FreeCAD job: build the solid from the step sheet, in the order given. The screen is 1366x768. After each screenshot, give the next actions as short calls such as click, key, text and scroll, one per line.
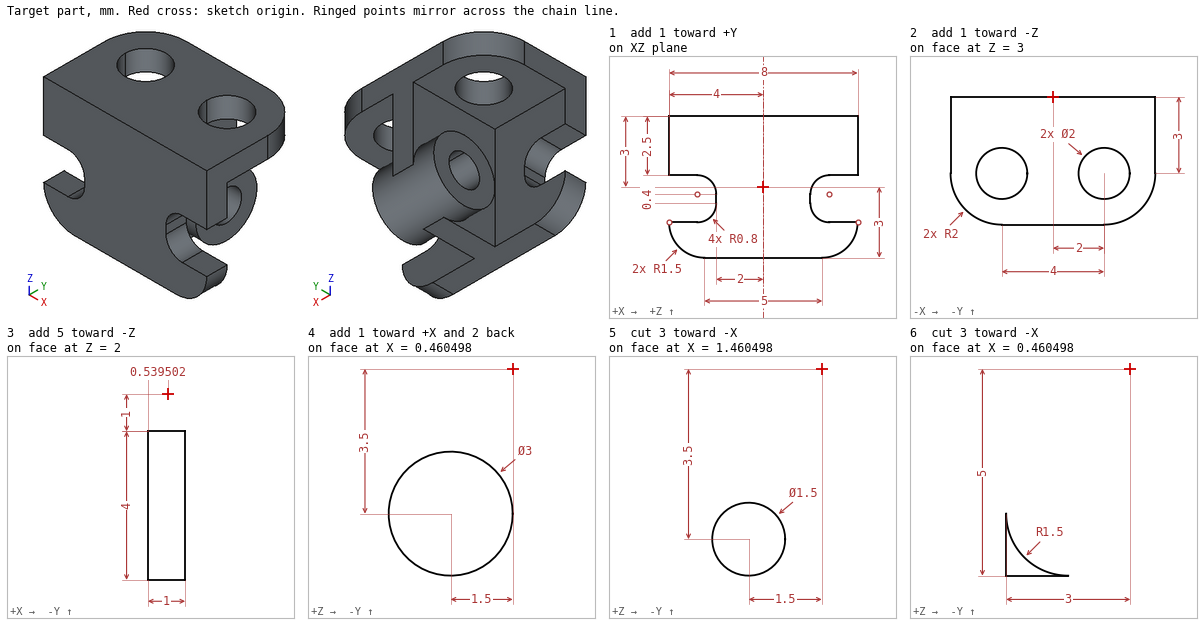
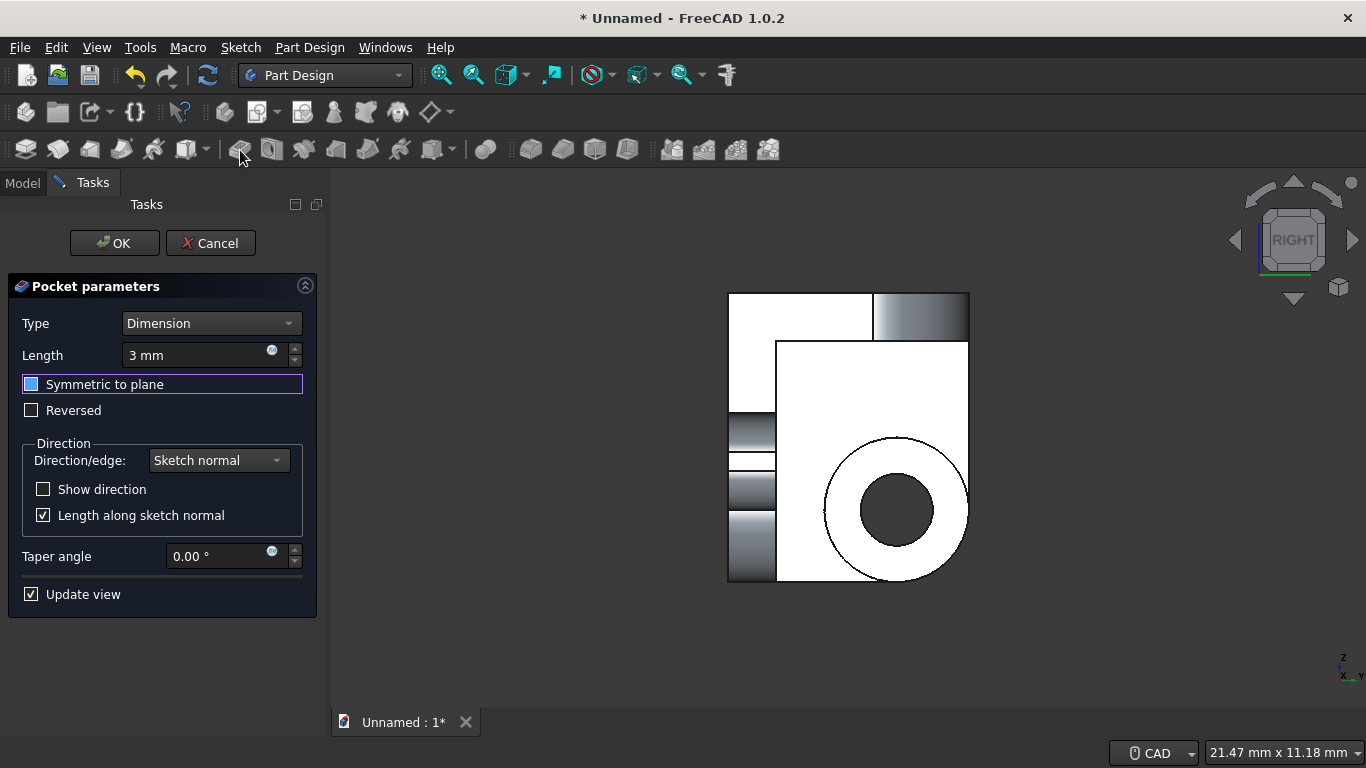
click(115, 243)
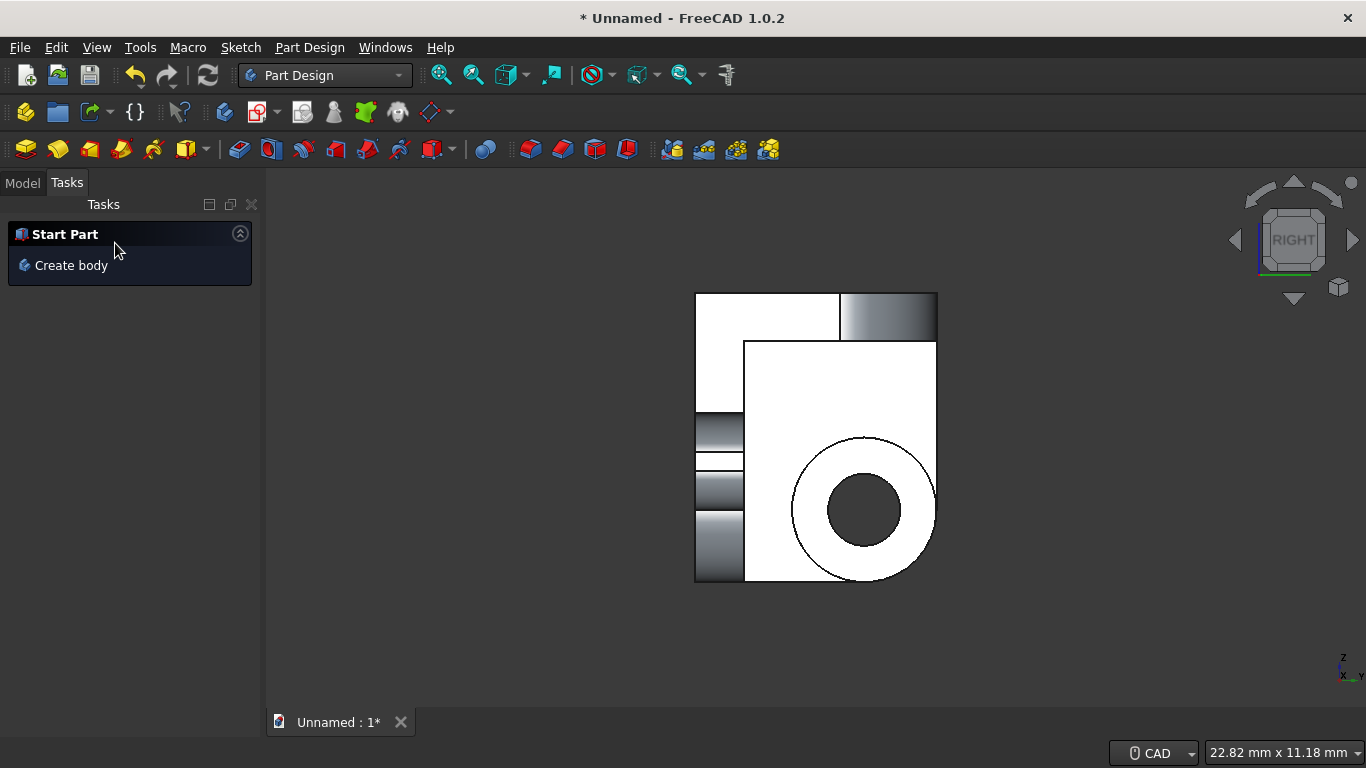
key(0)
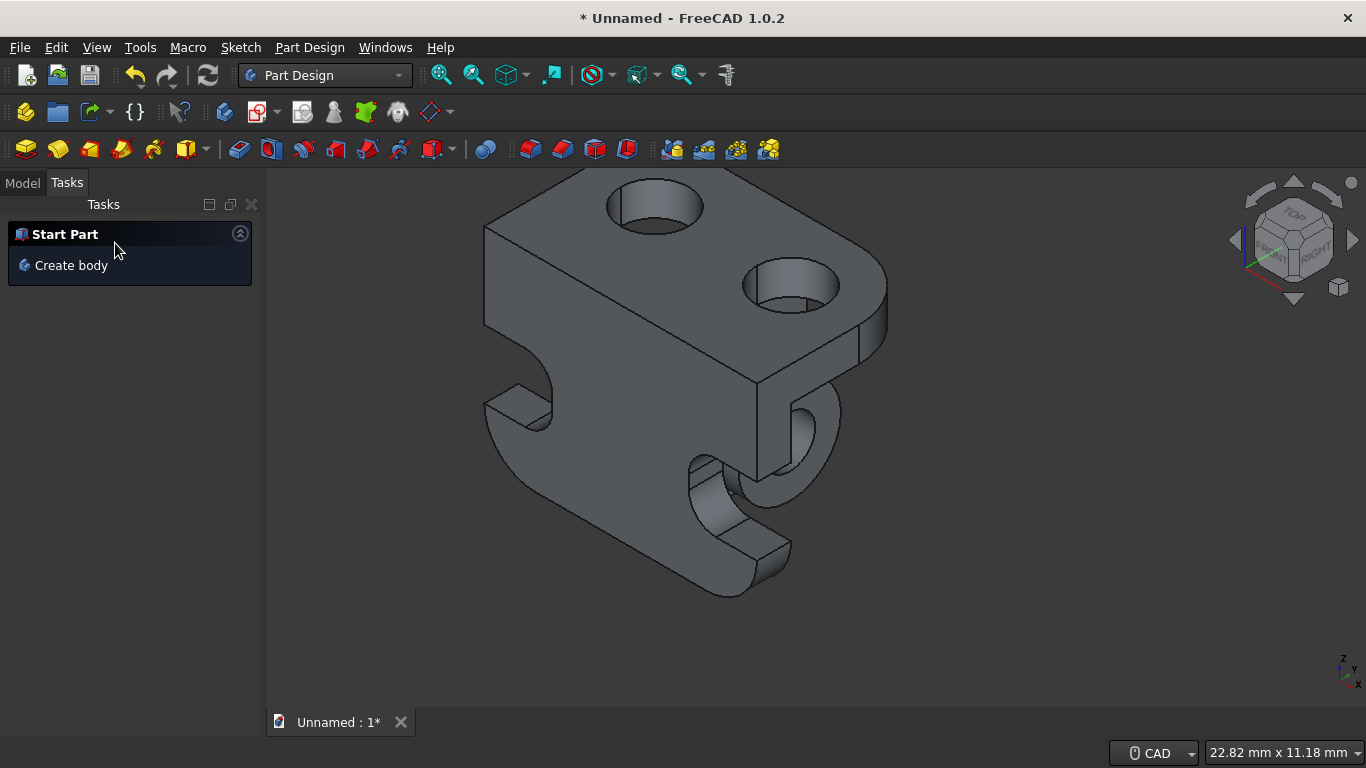
click(442, 76)